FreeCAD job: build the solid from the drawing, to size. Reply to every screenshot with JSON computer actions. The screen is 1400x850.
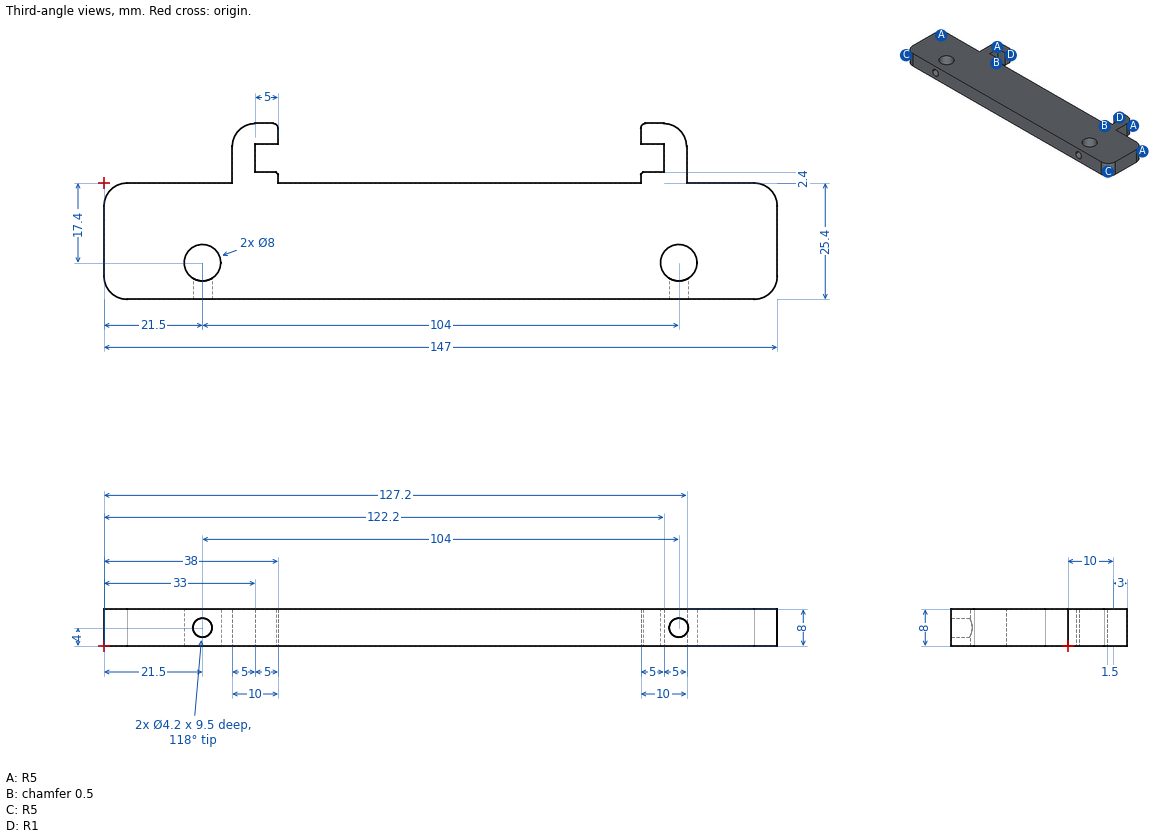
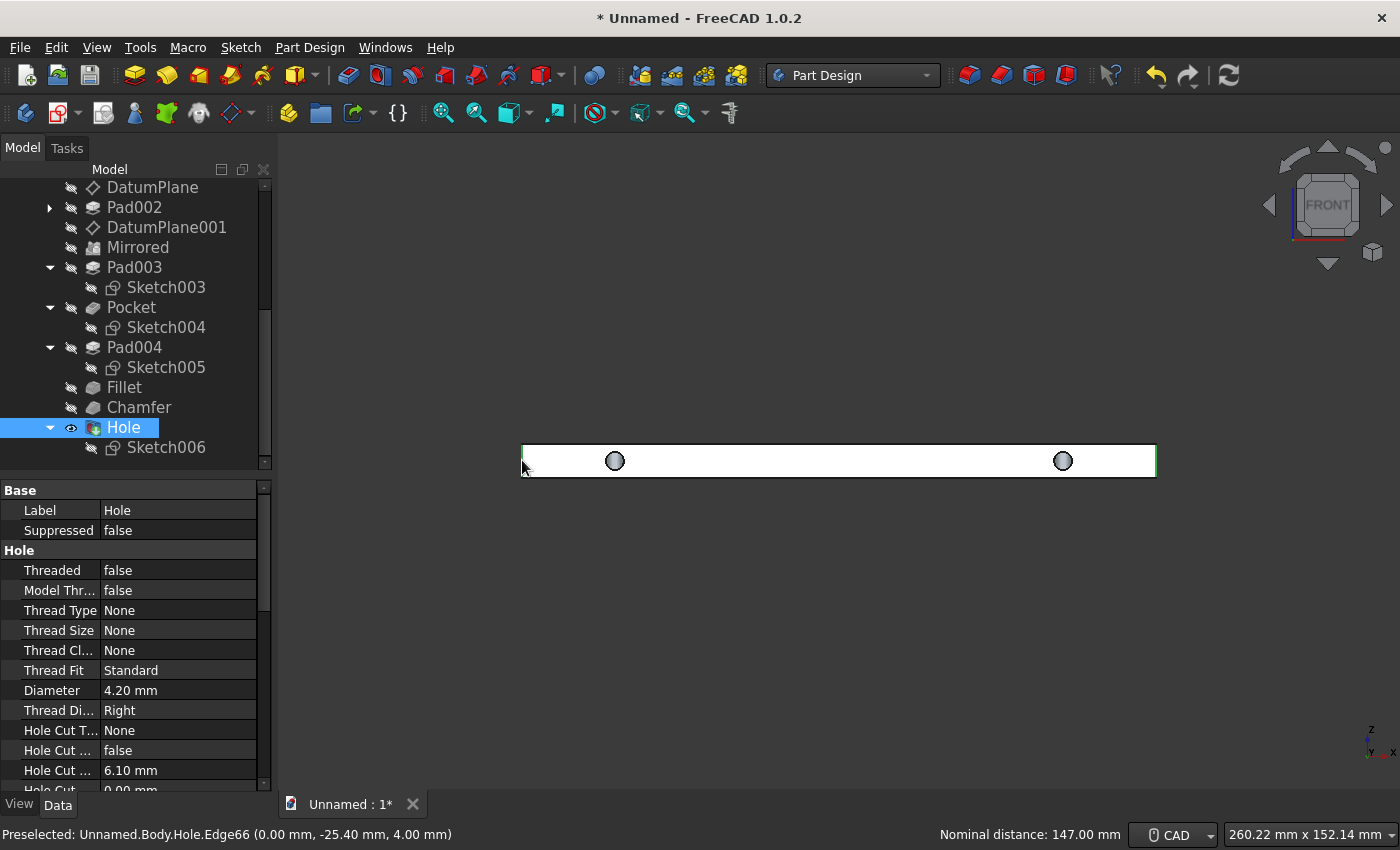
{"action": "left_click", "coordinate": [970, 76]}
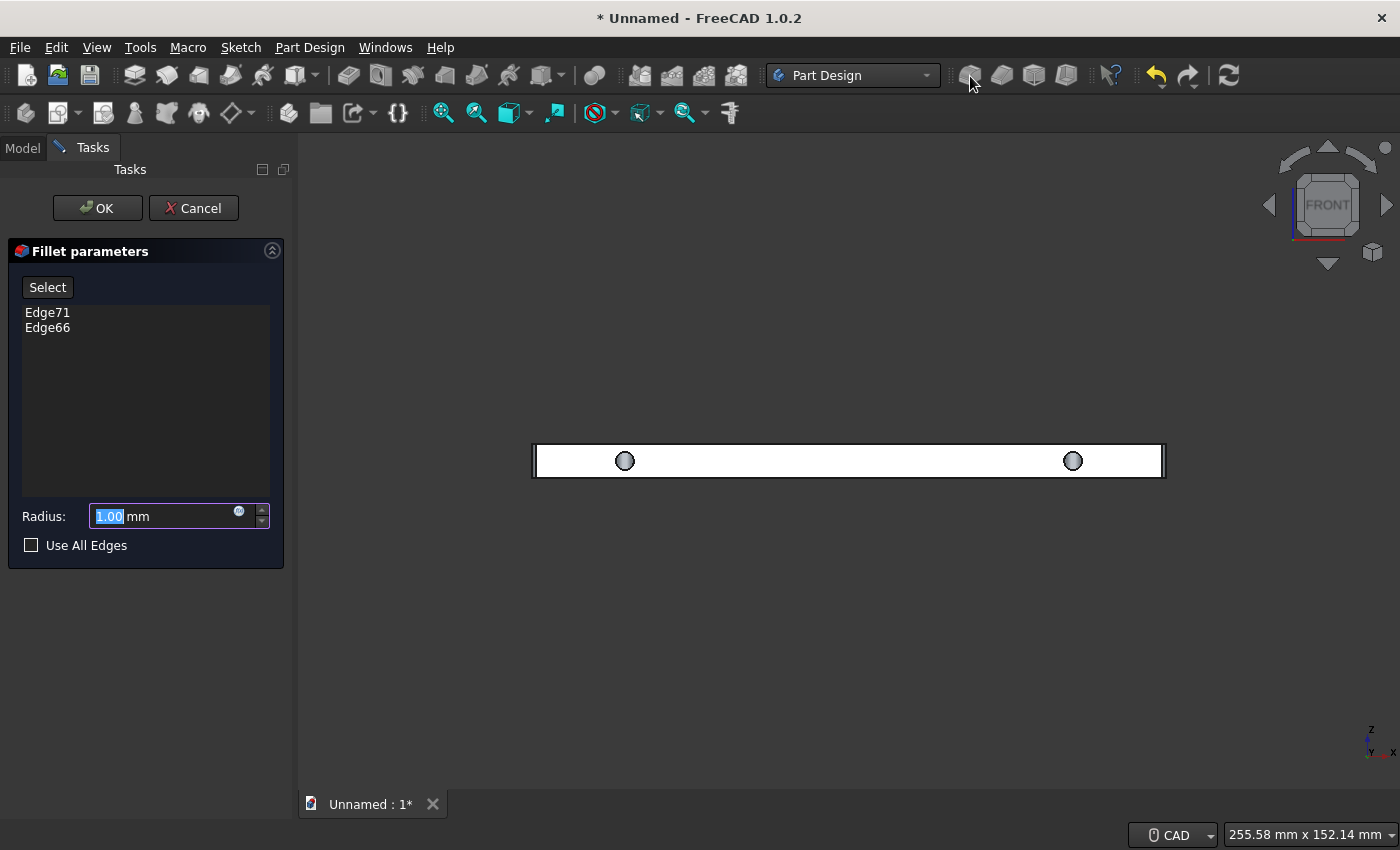
{"action": "type", "text": "5"}
{"action": "key", "text": "Tab"}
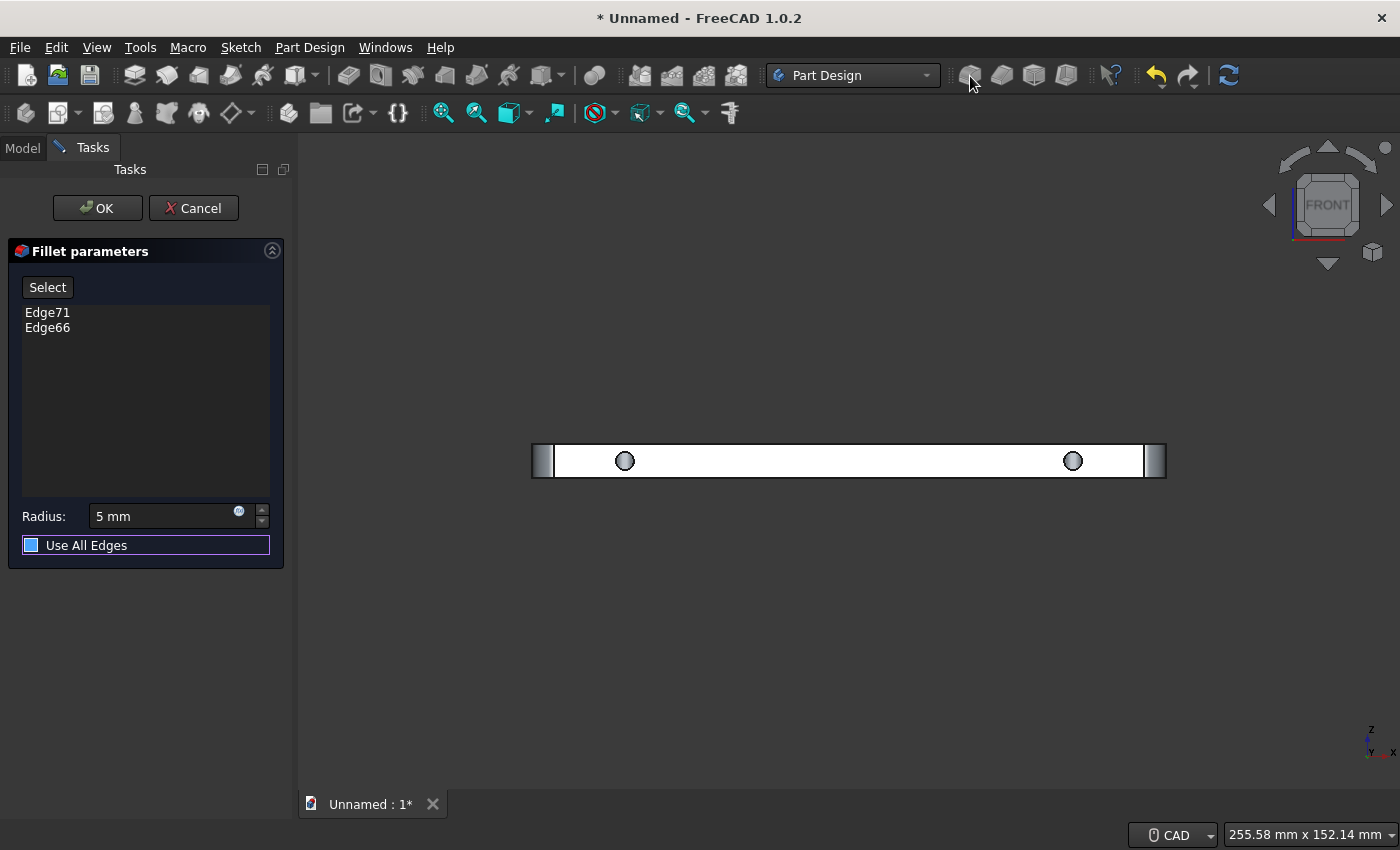
{"action": "left_click", "coordinate": [98, 208]}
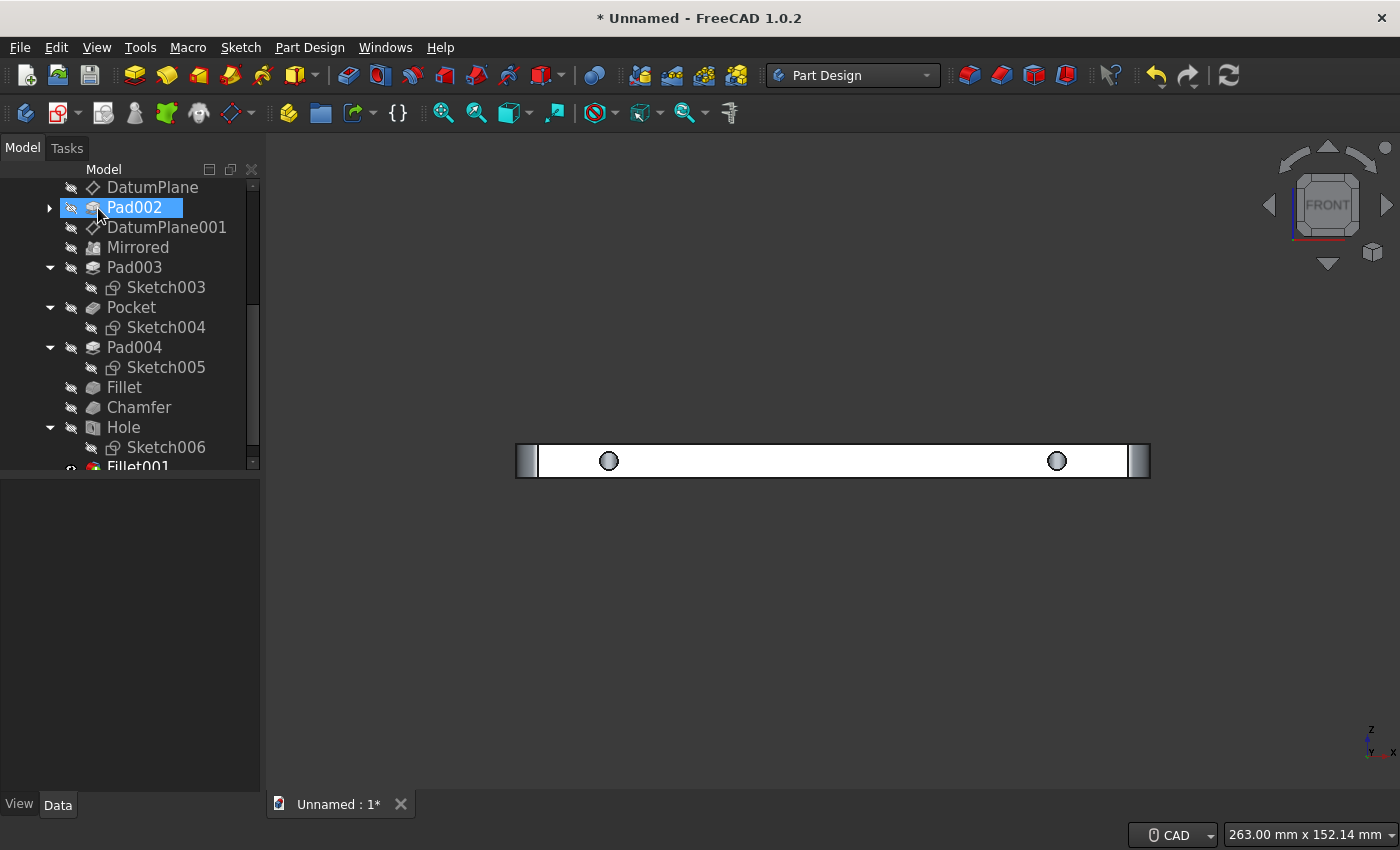
{"action": "key", "text": "0"}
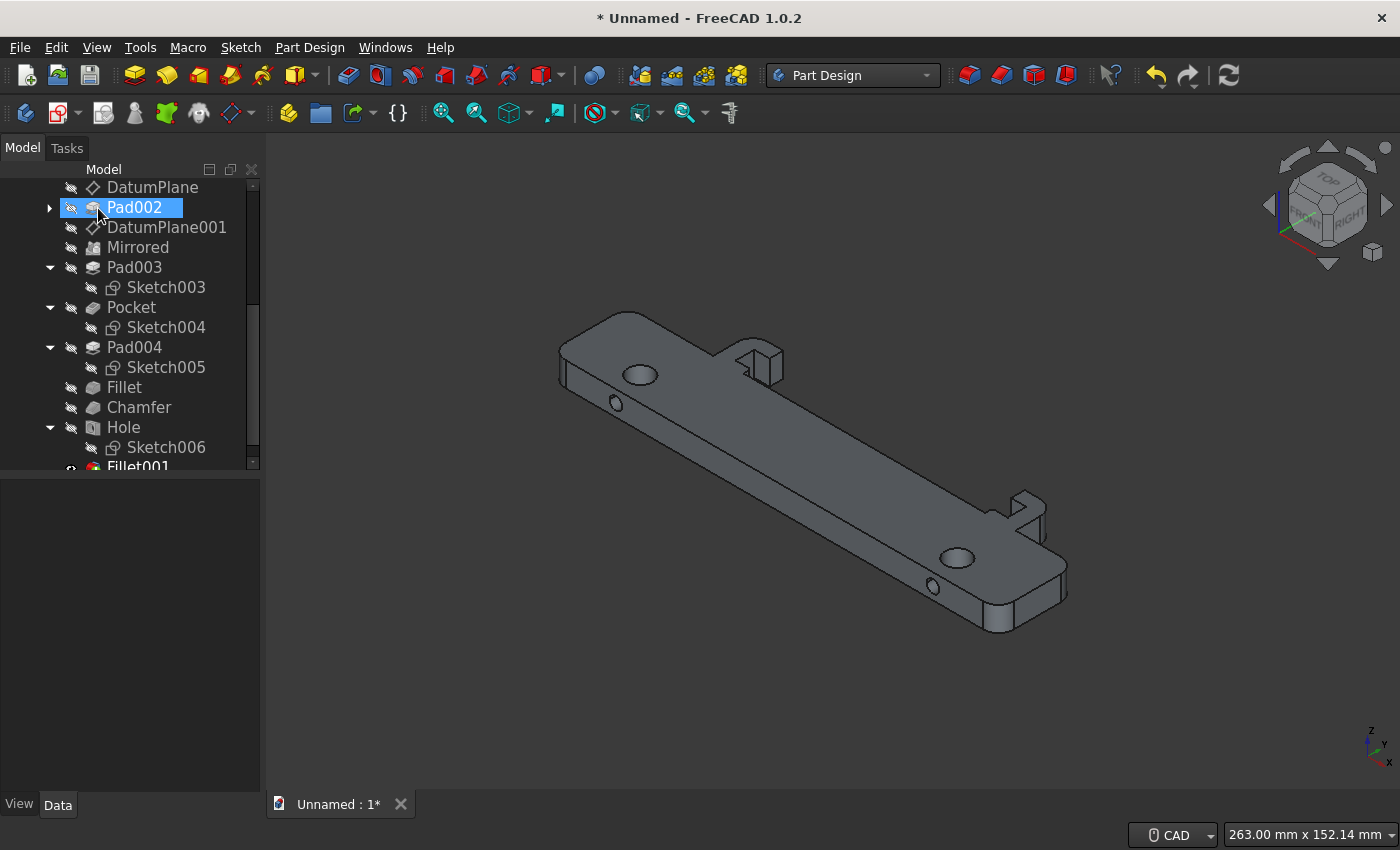
{"action": "key", "text": "2"}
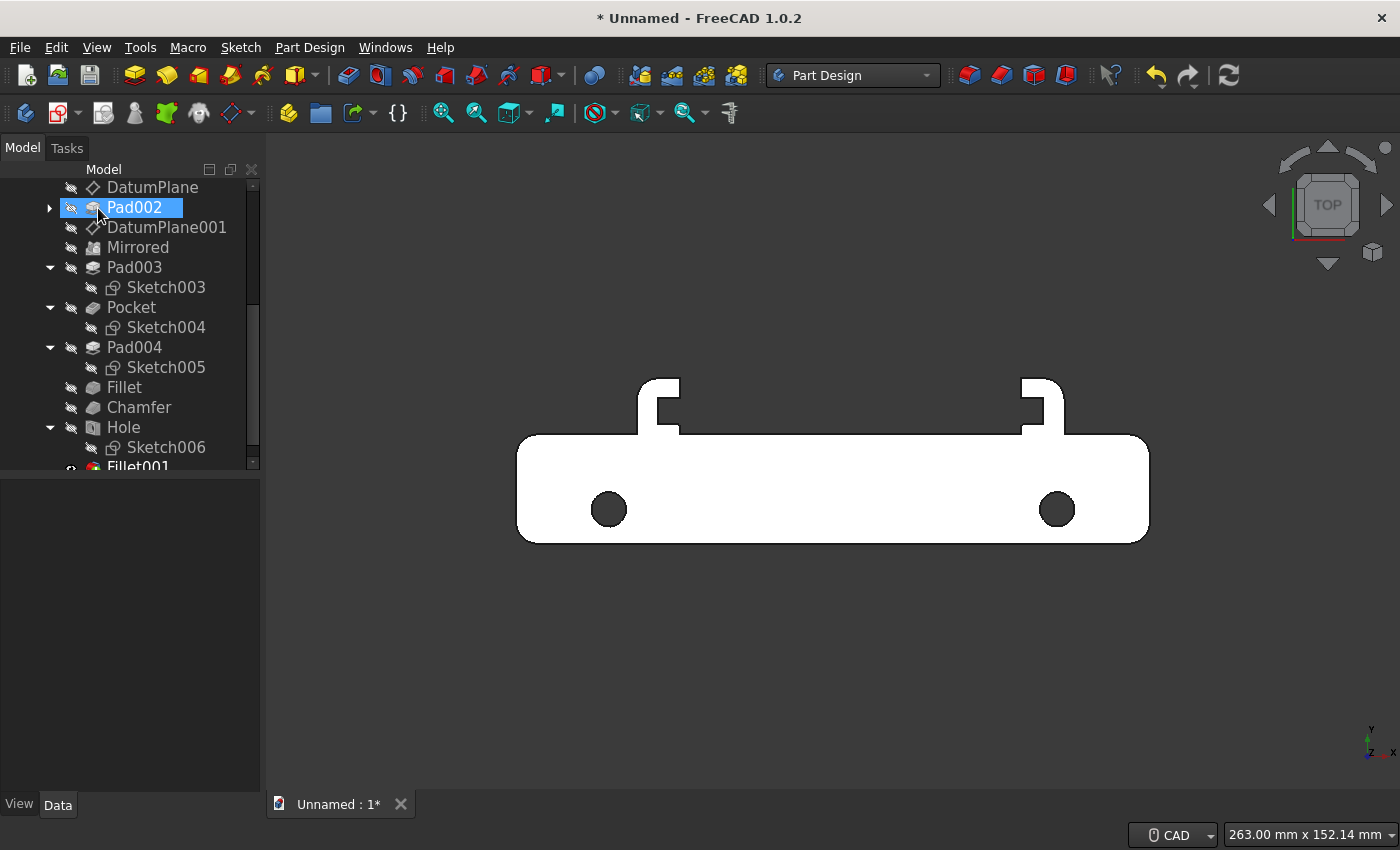
{"action": "key", "text": "1"}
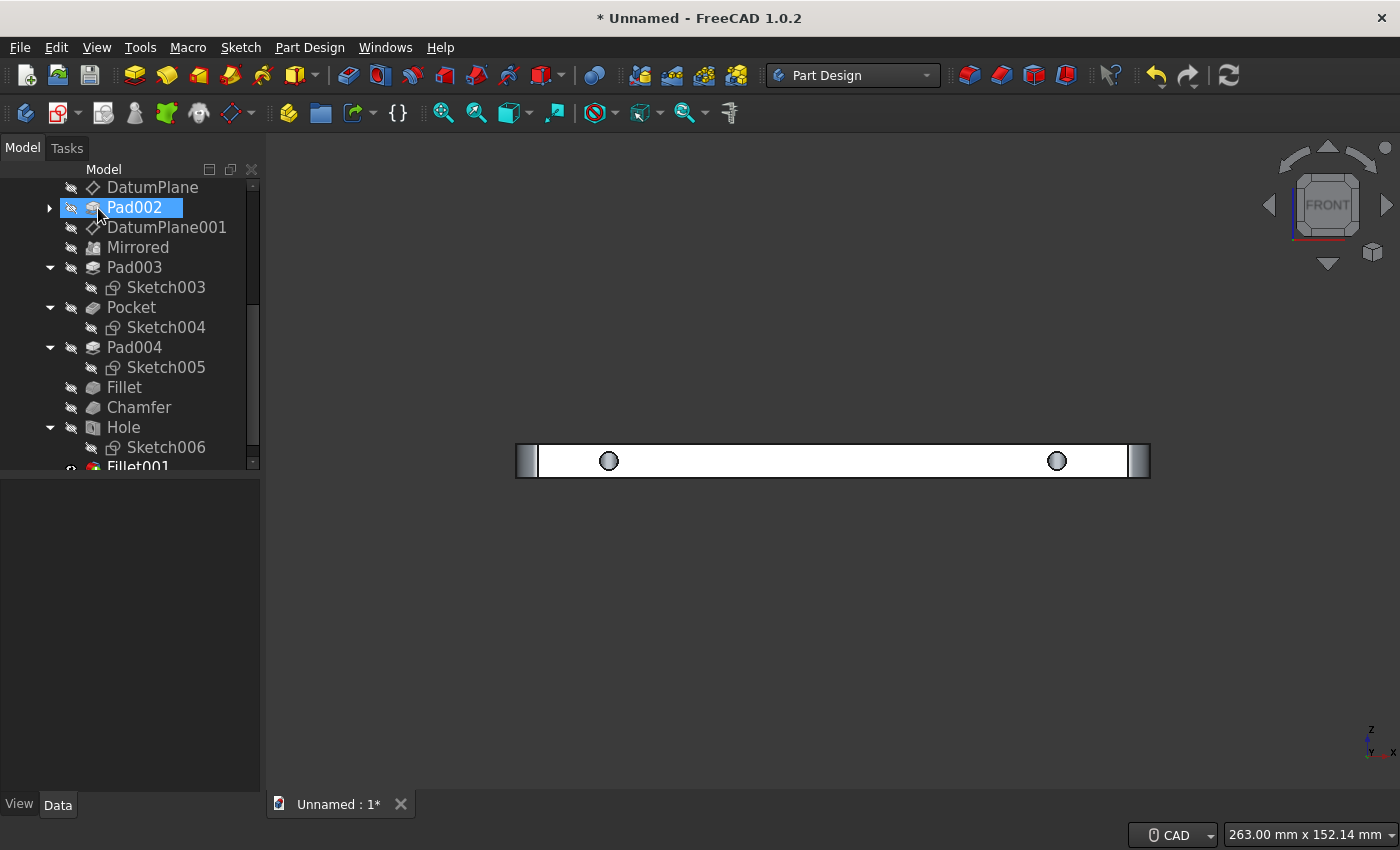
{"action": "key", "text": "3"}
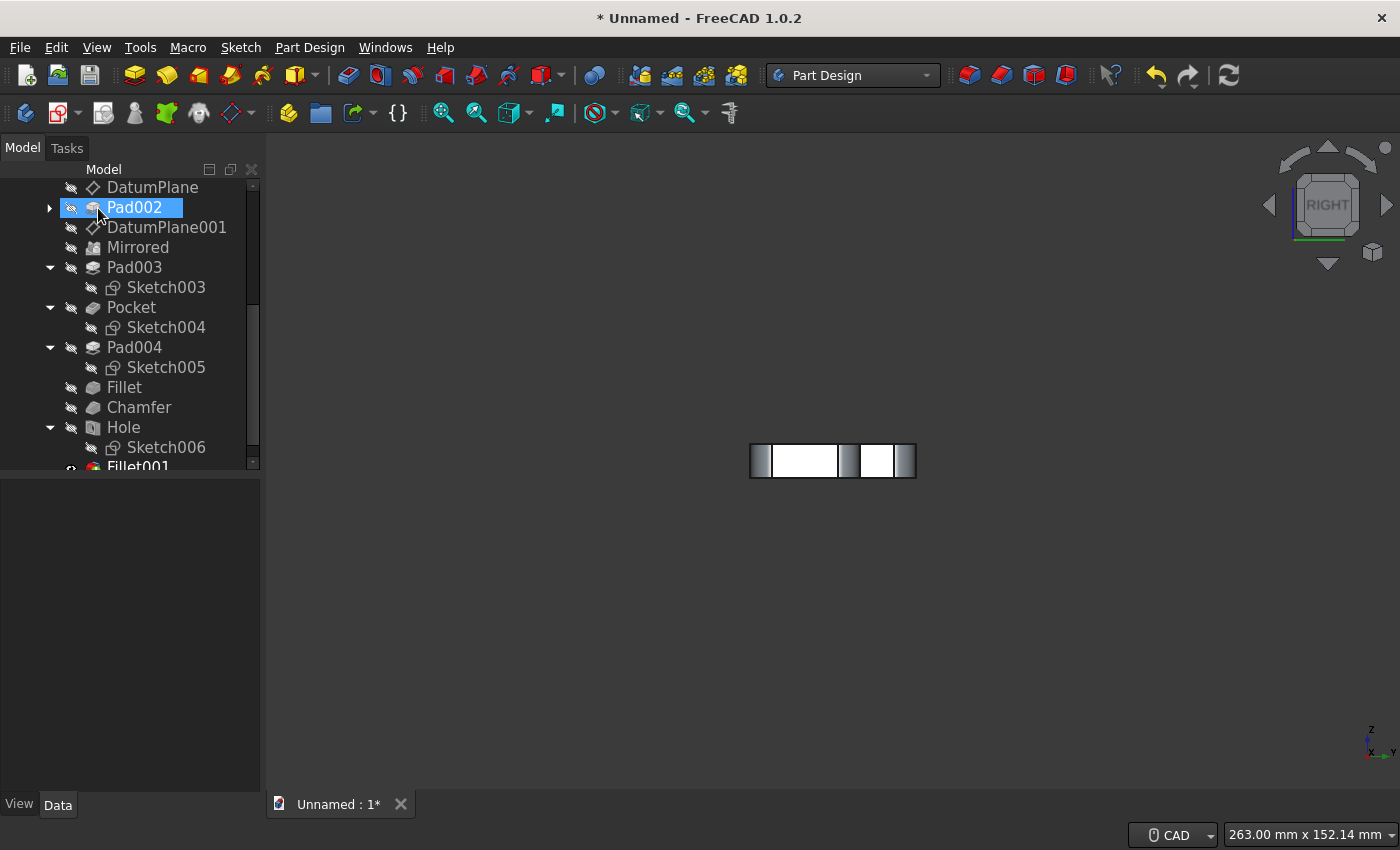
{"action": "left_click", "coordinate": [444, 114]}